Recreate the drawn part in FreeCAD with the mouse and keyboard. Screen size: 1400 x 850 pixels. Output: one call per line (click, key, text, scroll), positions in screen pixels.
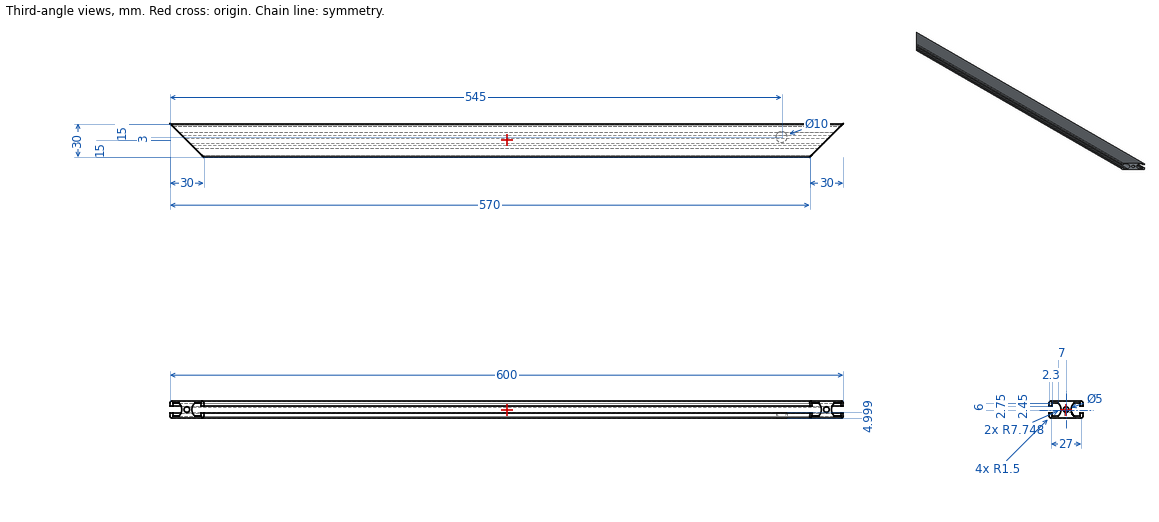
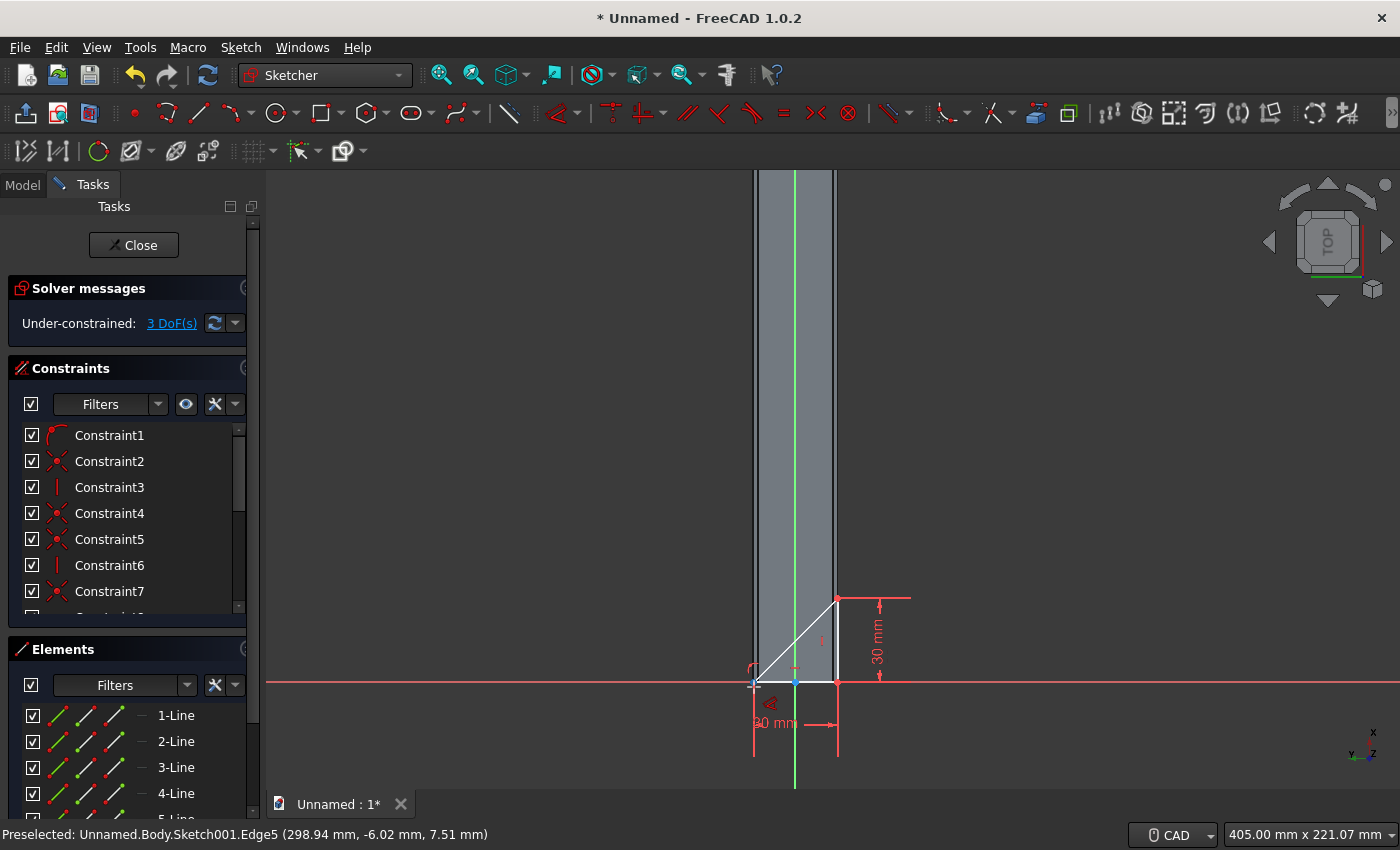
click(754, 682)
click(765, 648)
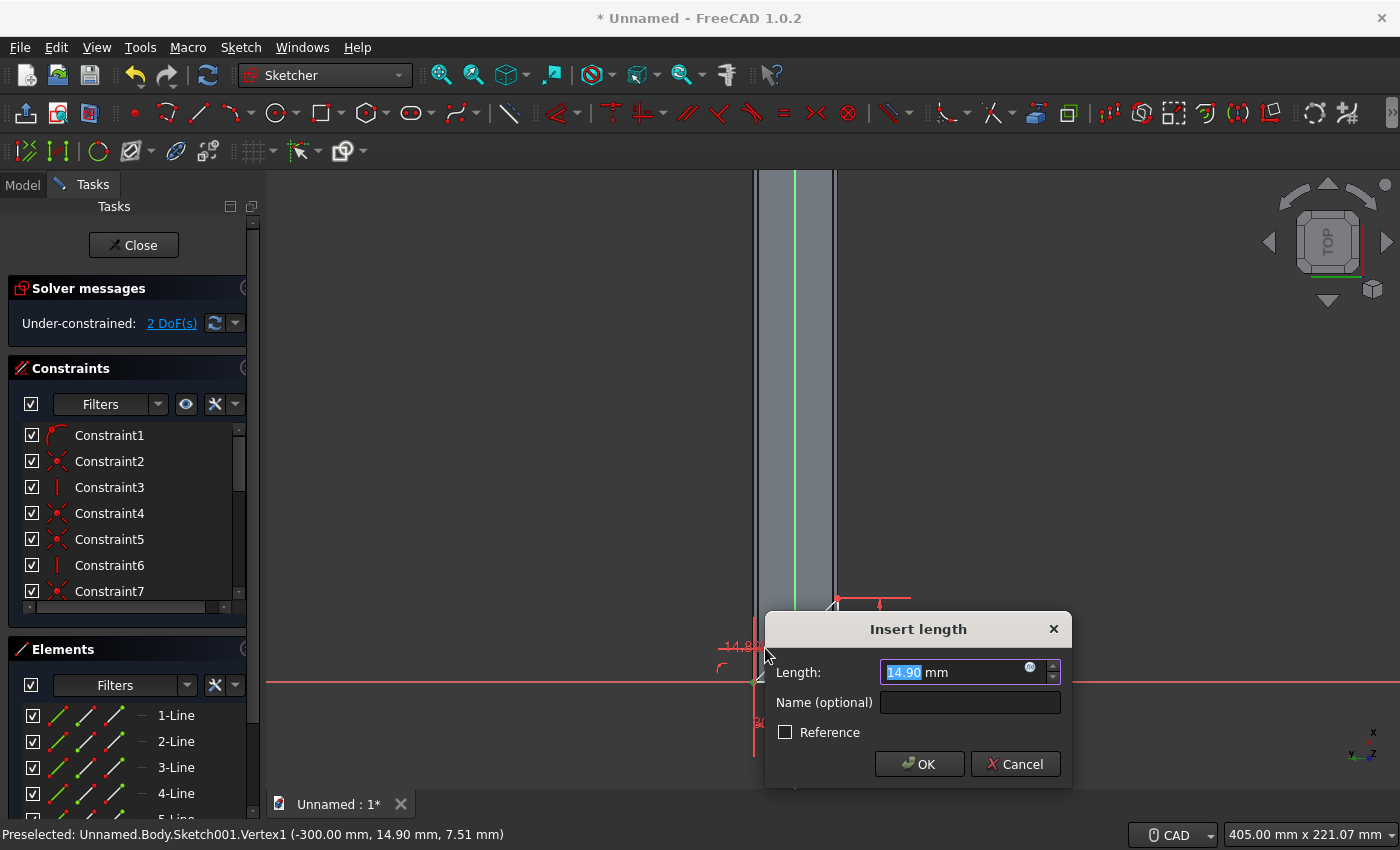
text(15)
key(Return)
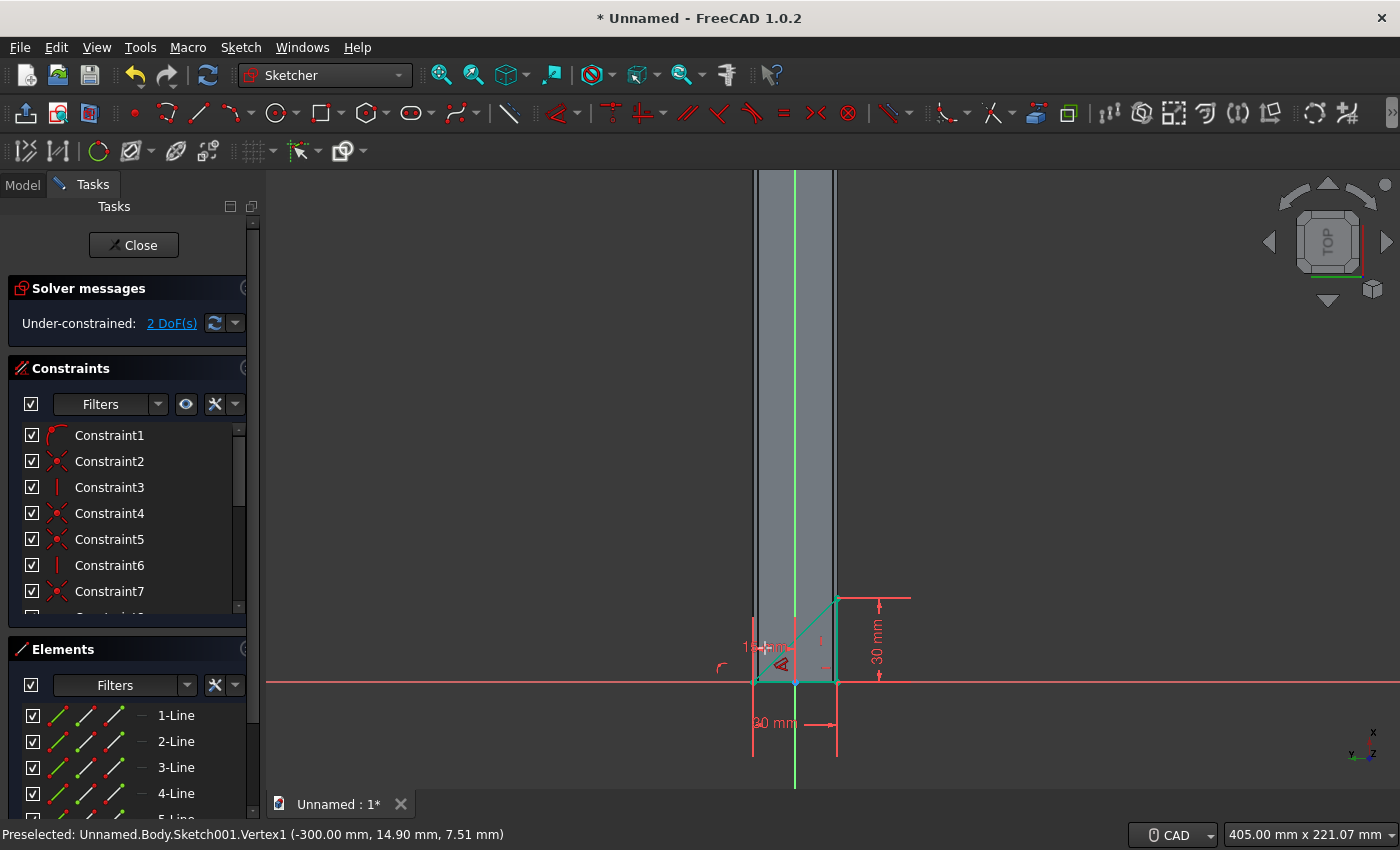
scroll(754, 688, down, 7)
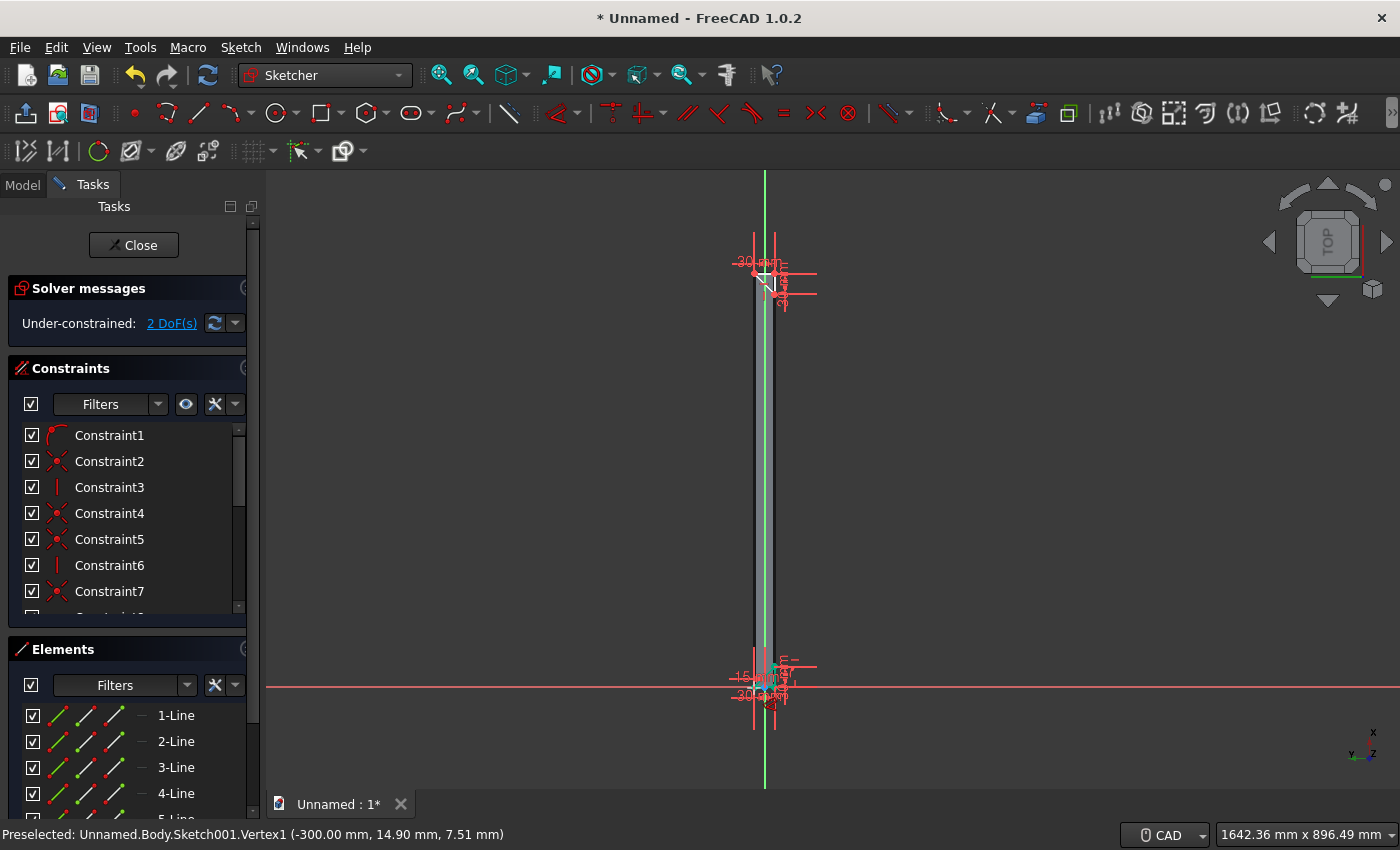
scroll(775, 294, up, 7)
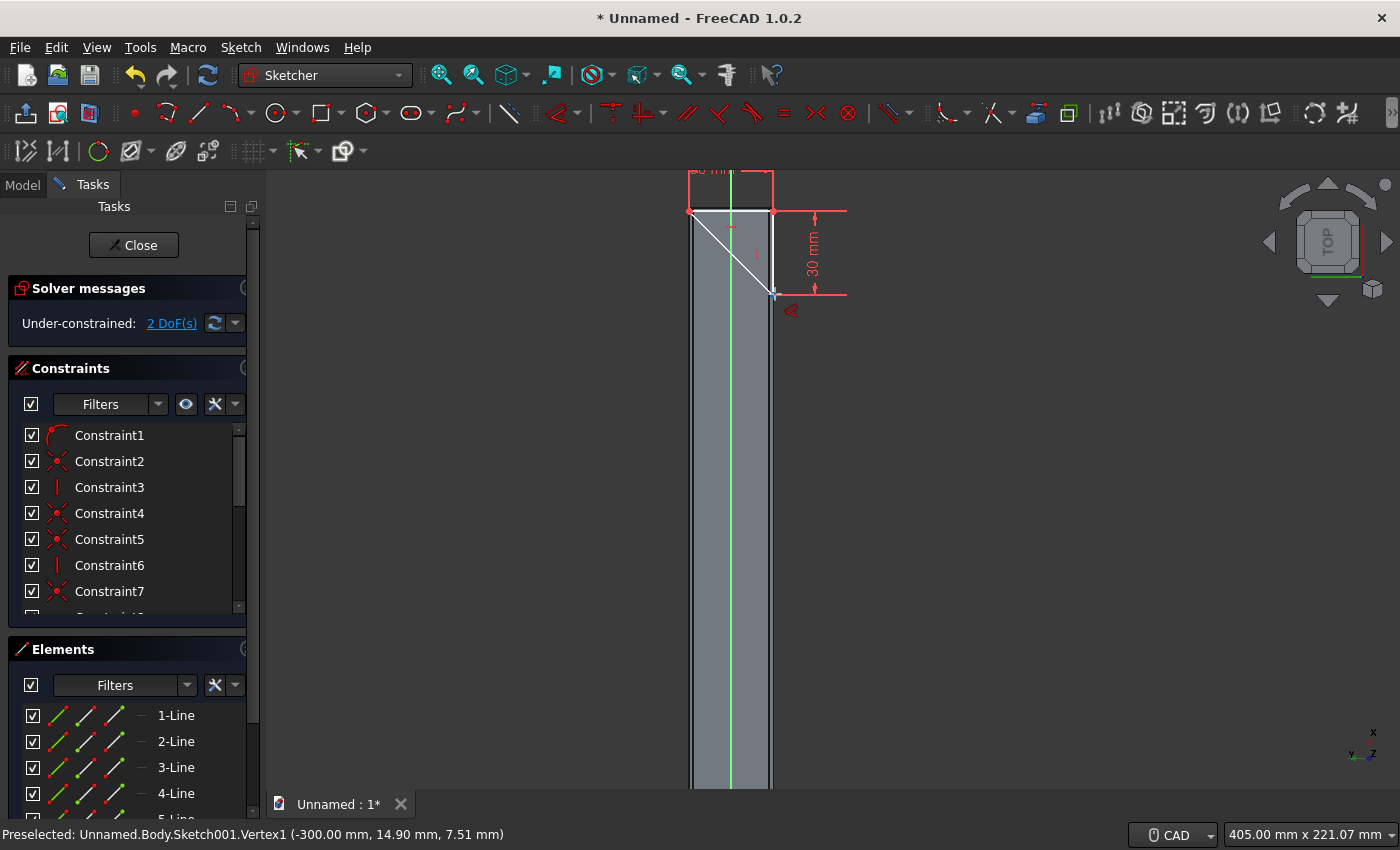
click(773, 295)
click(752, 261)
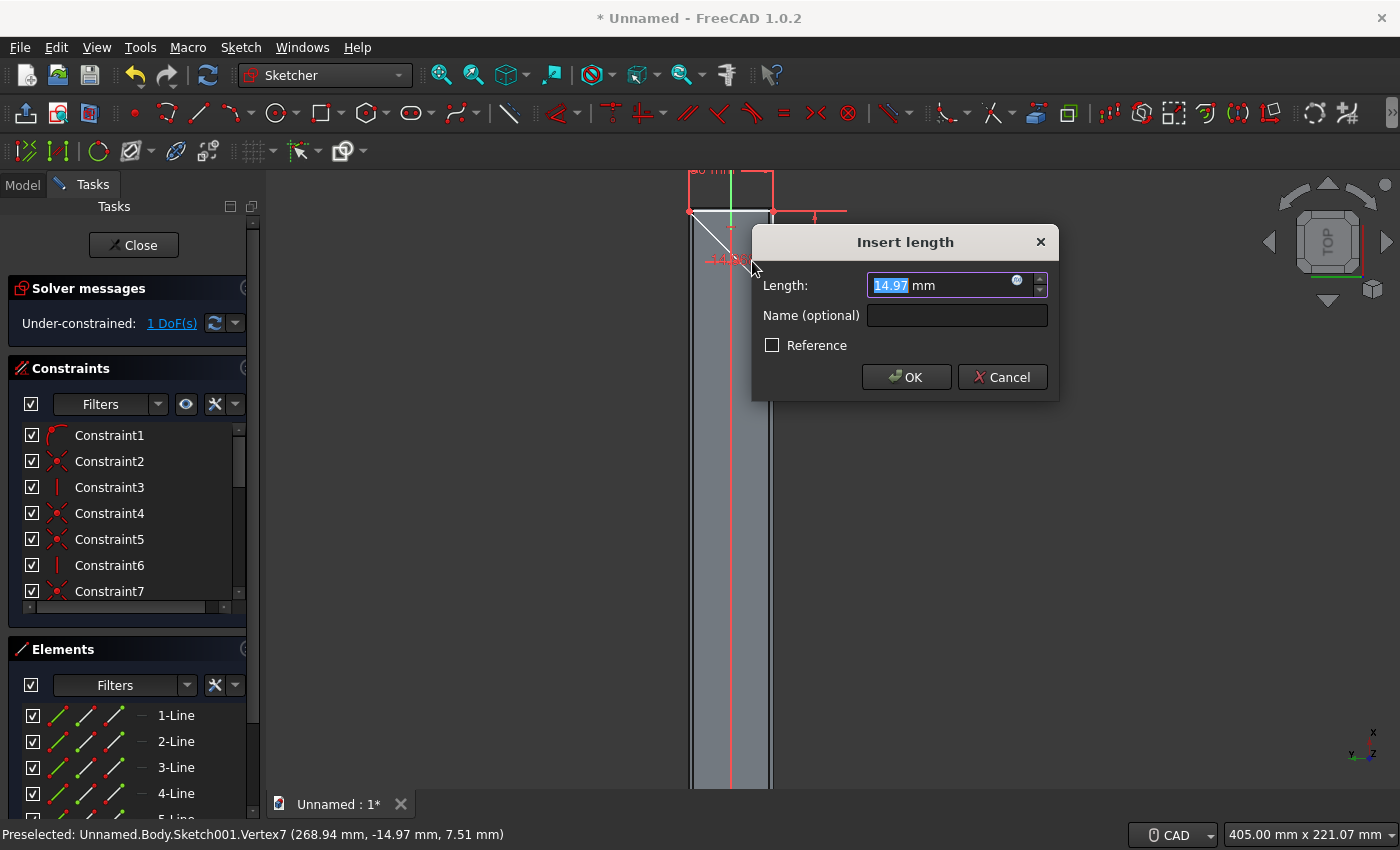
text(15)
key(Return)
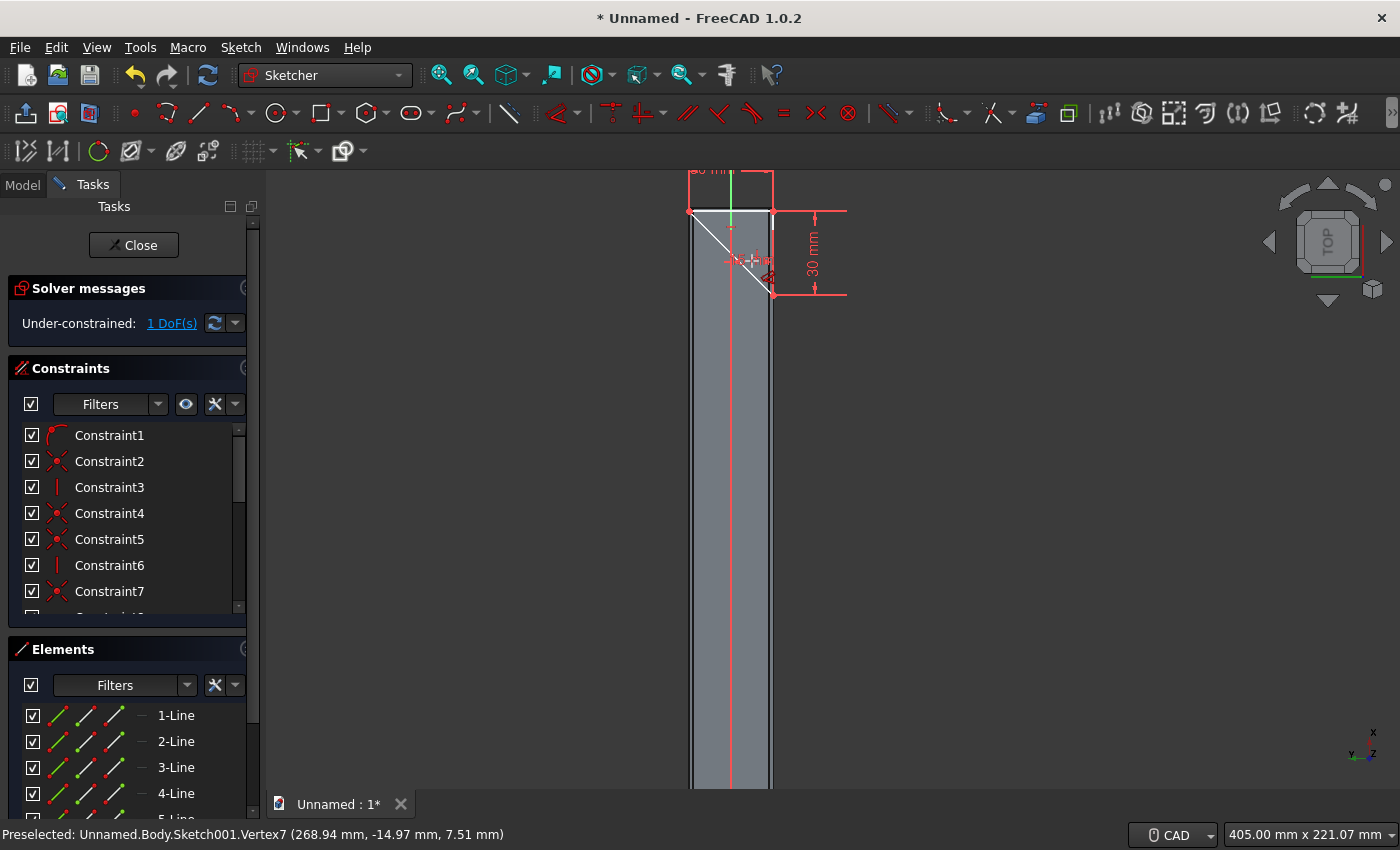
scroll(775, 293, down, 7)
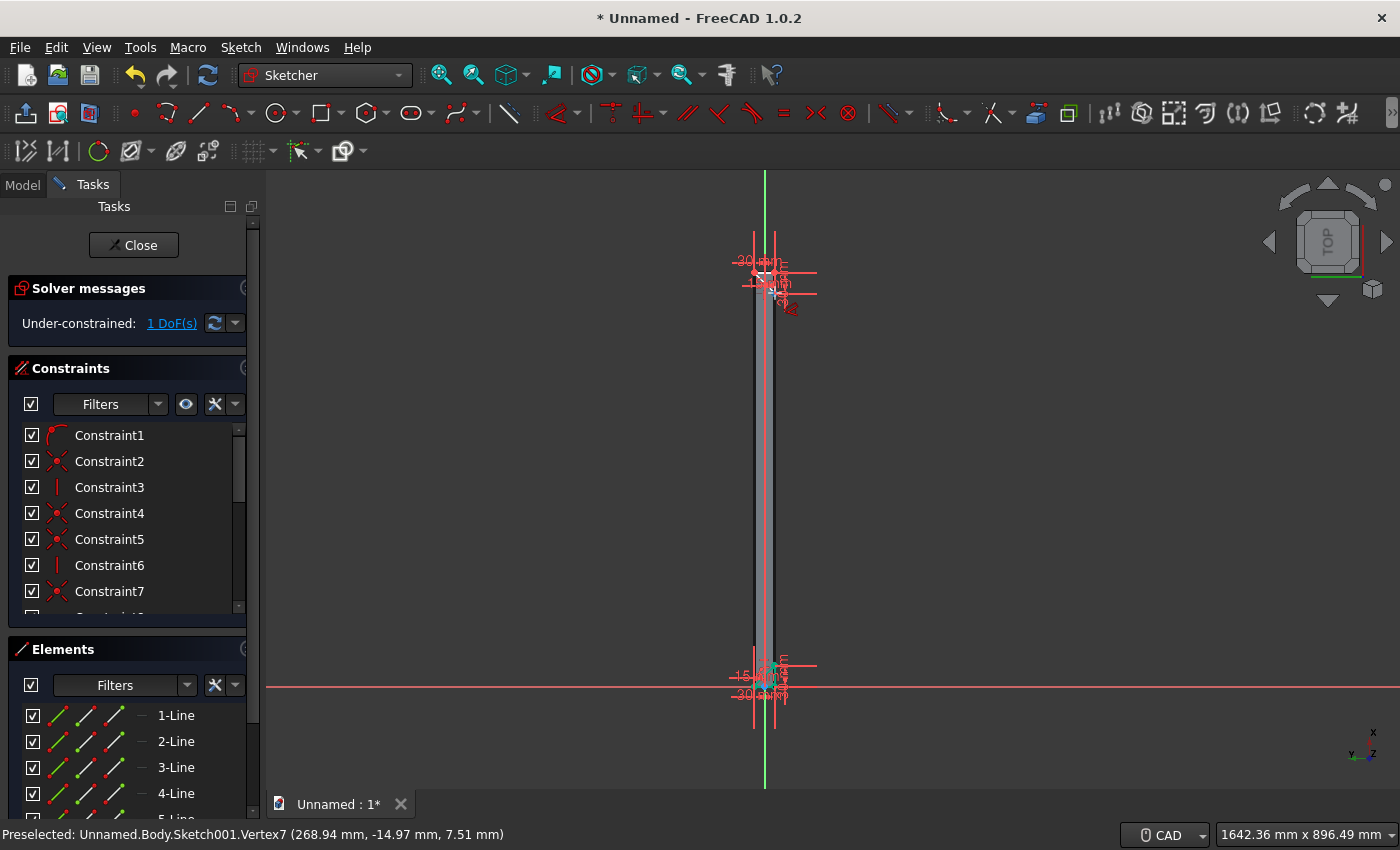
click(775, 294)
click(809, 490)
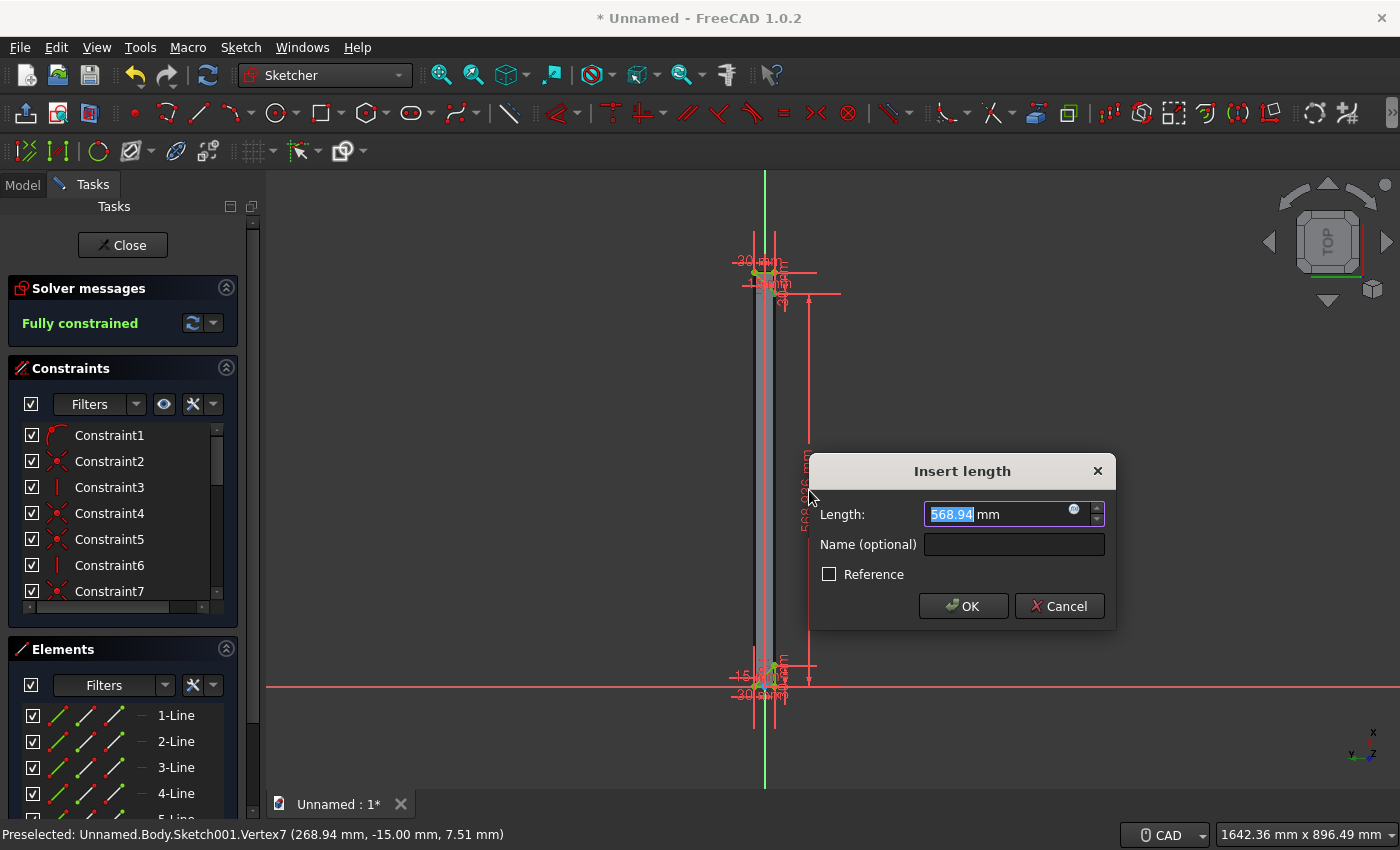
text(570)
key(Return)
key(Escape)